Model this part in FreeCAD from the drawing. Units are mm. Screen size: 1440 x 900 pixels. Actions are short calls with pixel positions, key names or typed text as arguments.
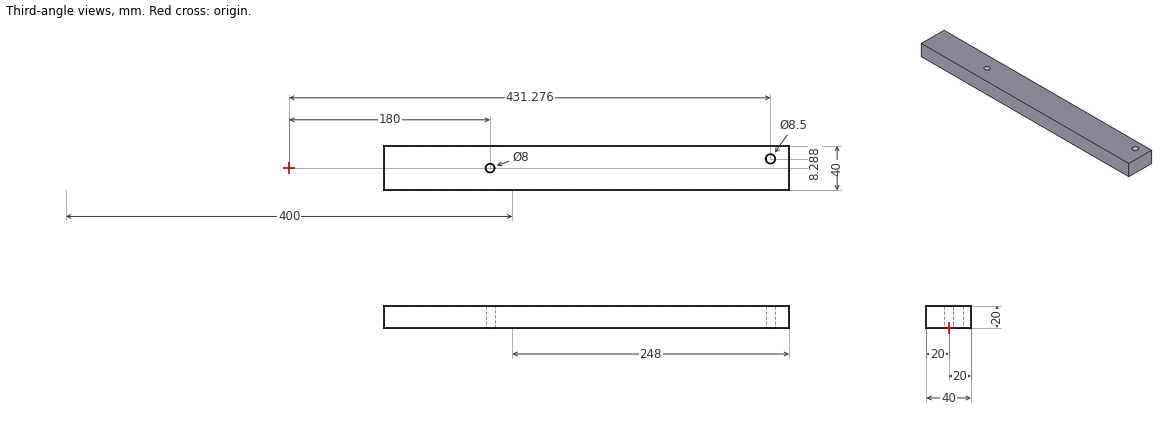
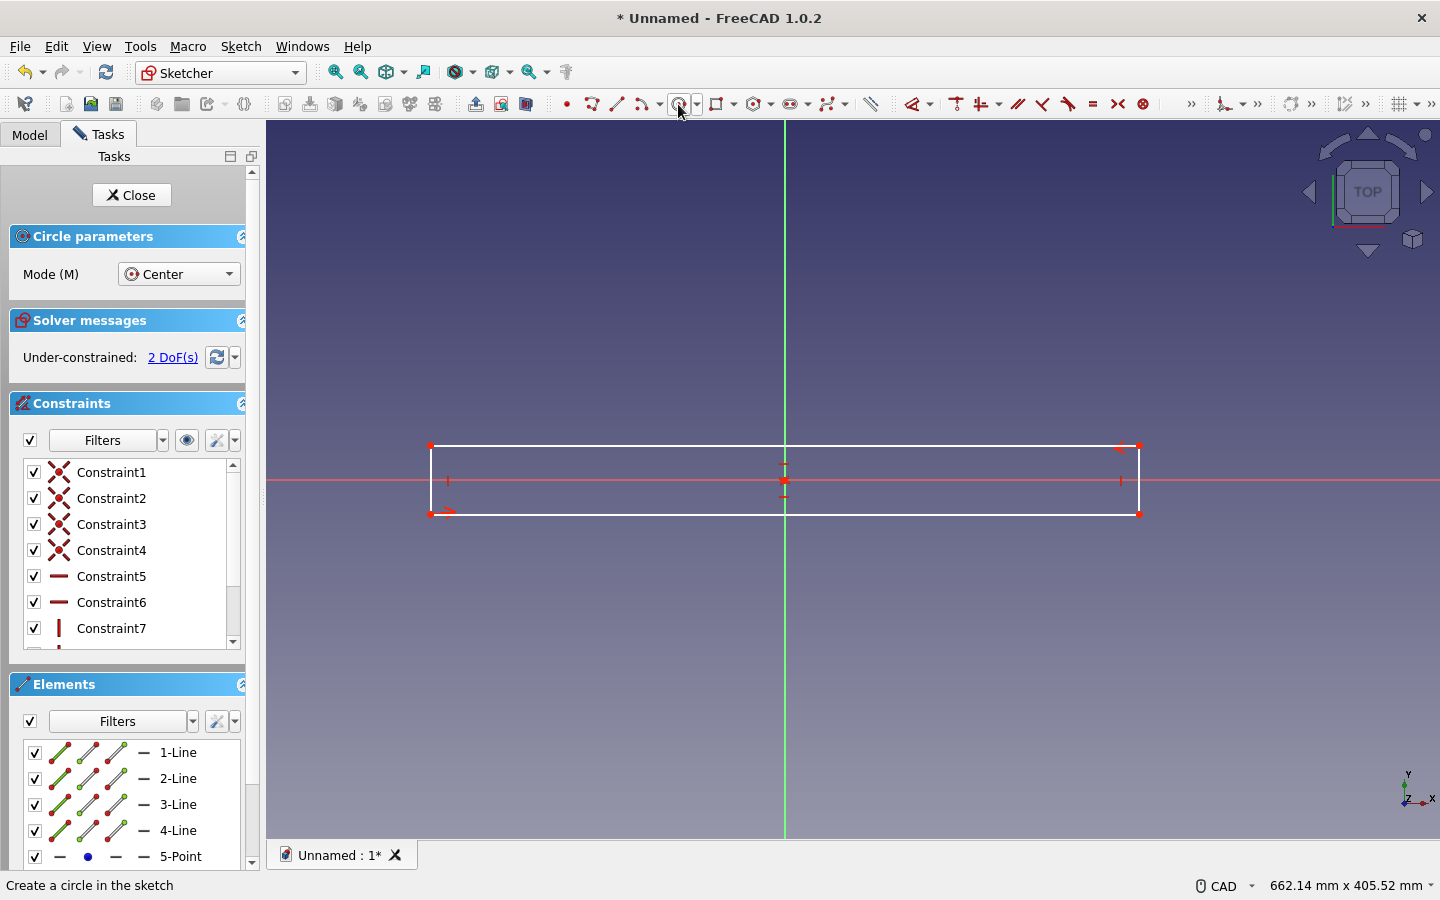
scroll(1104, 480, up, 6)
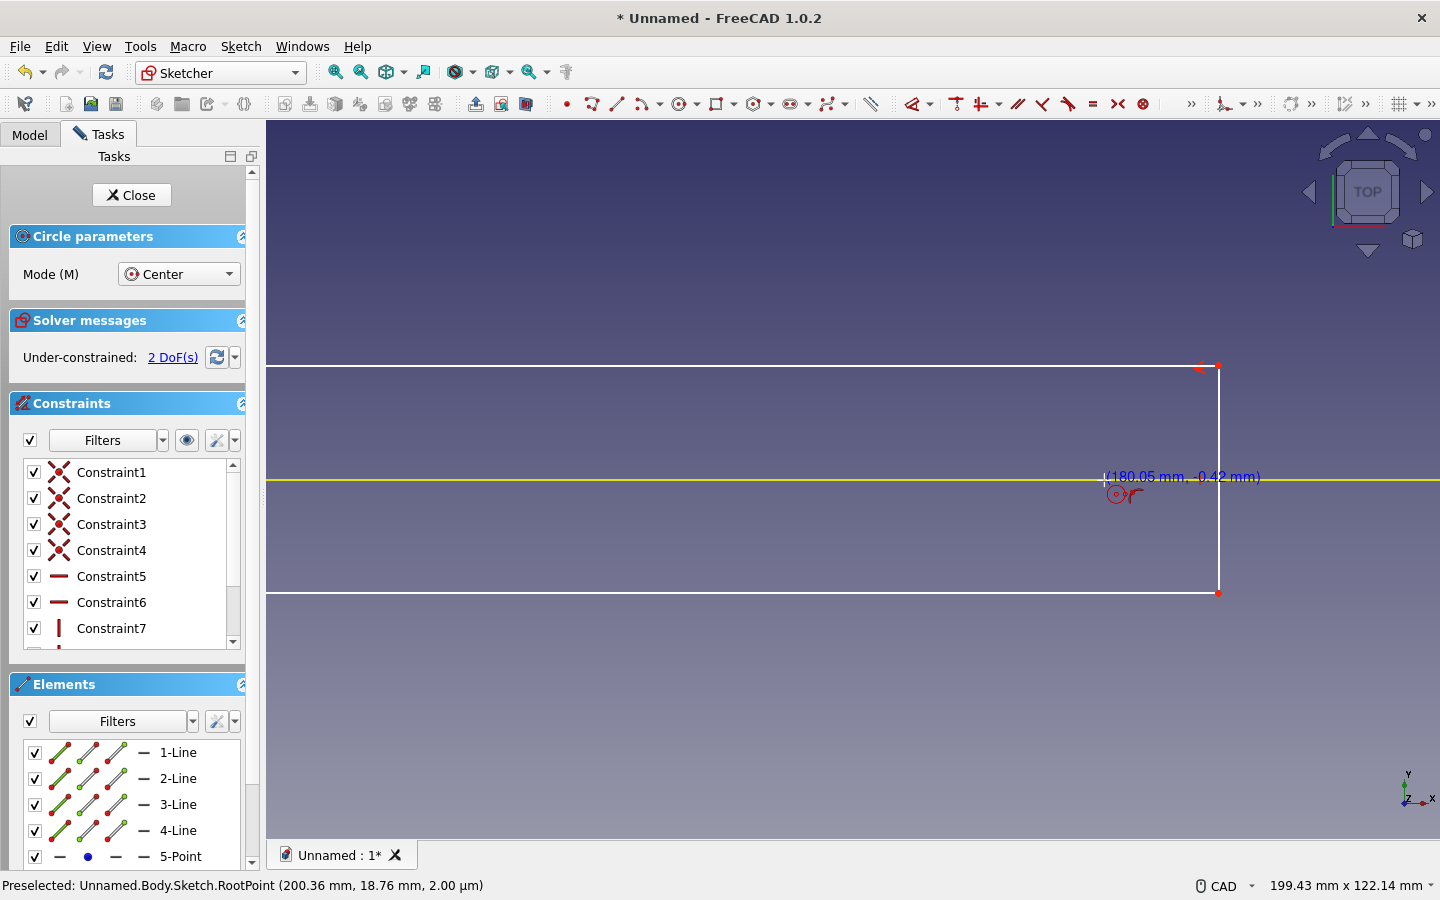
click(1102, 480)
click(1119, 463)
key(Escape)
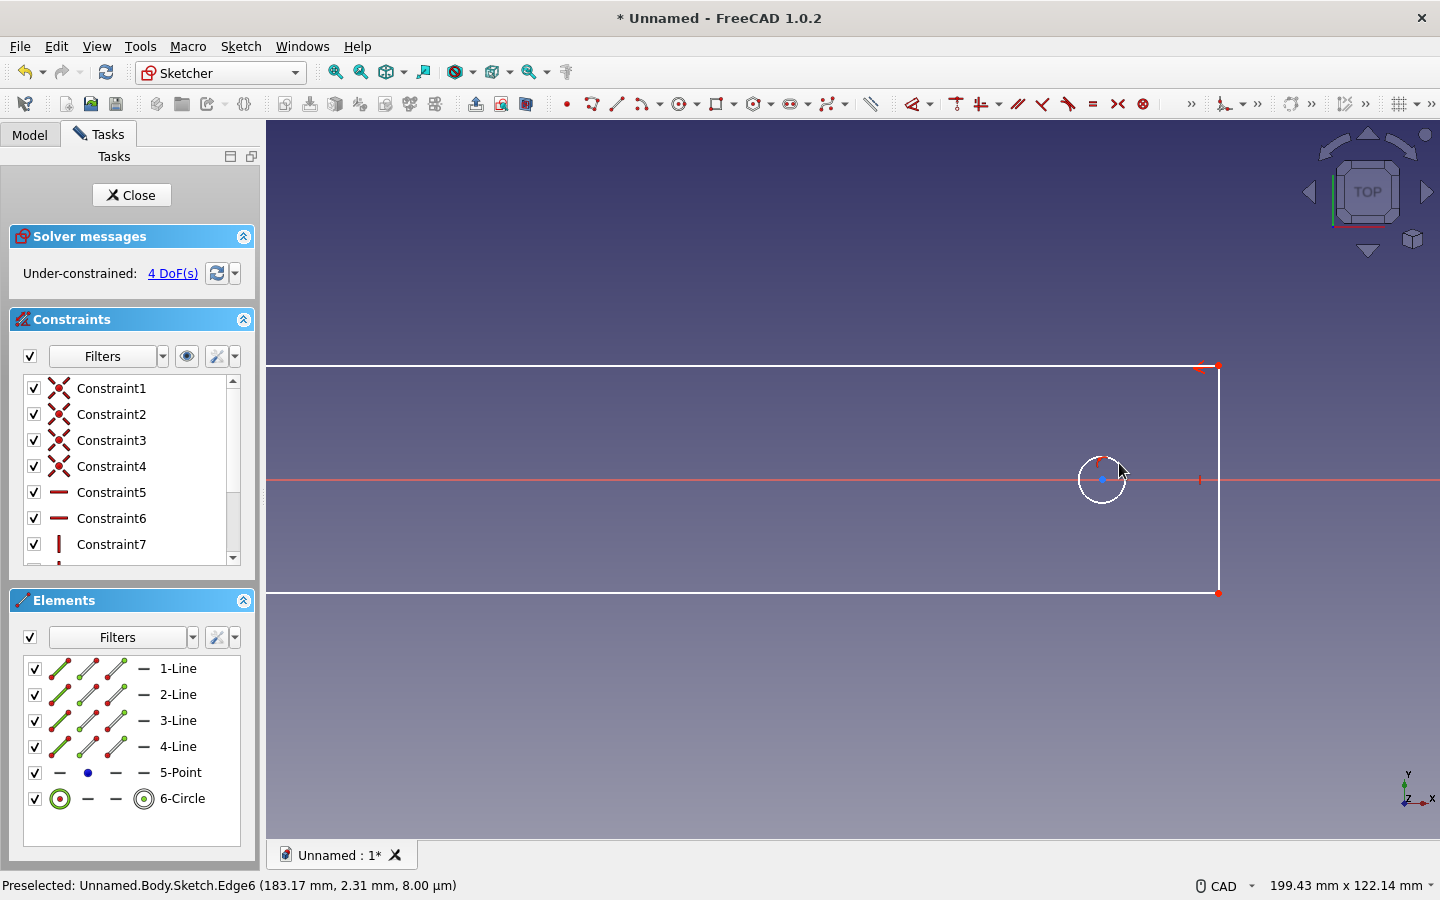
click(1118, 463)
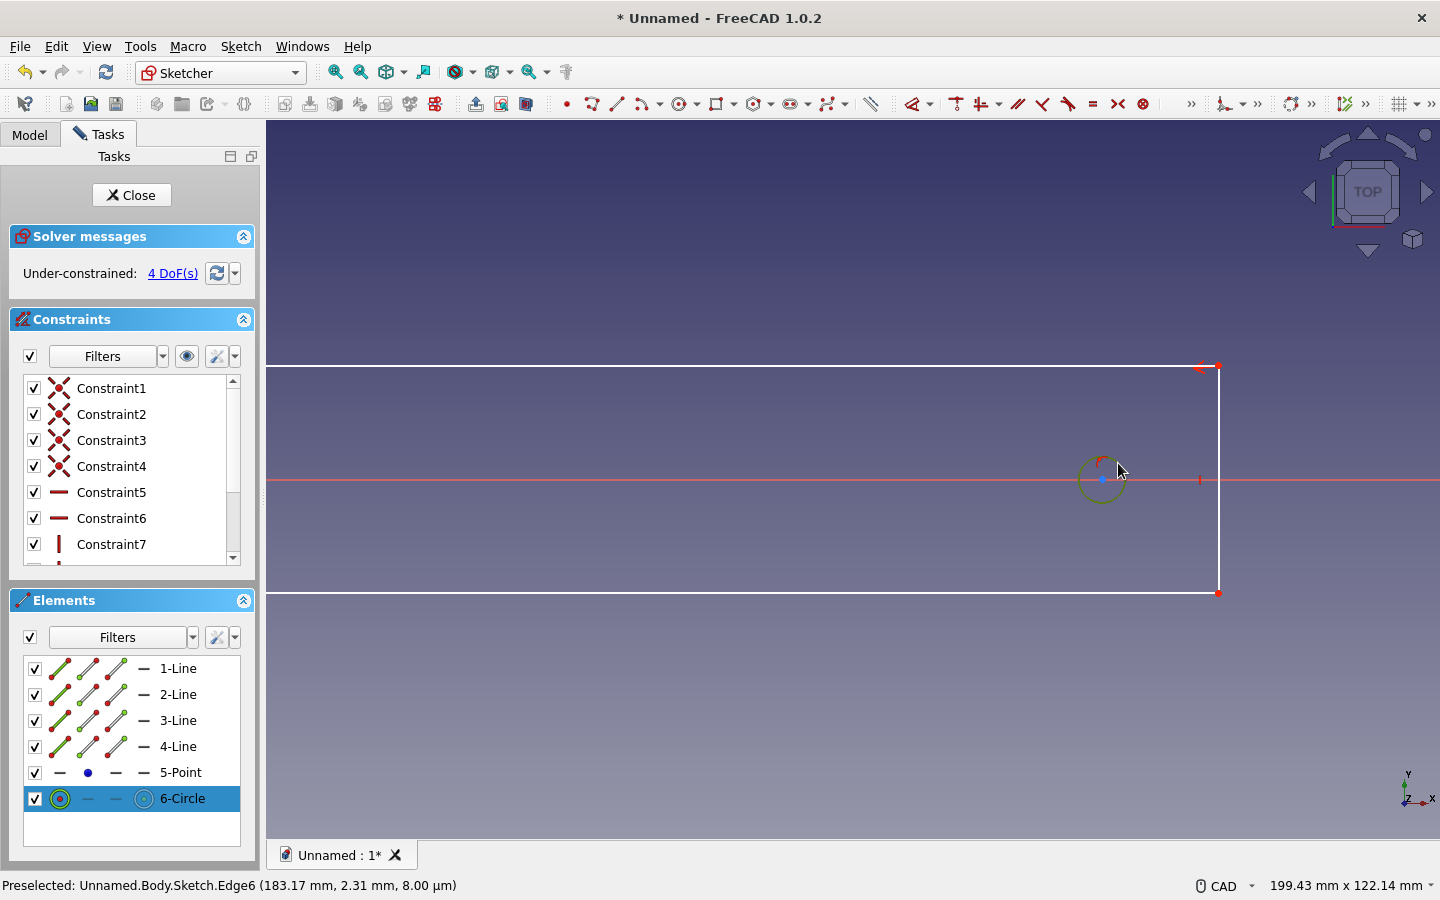
key(k)
key(o)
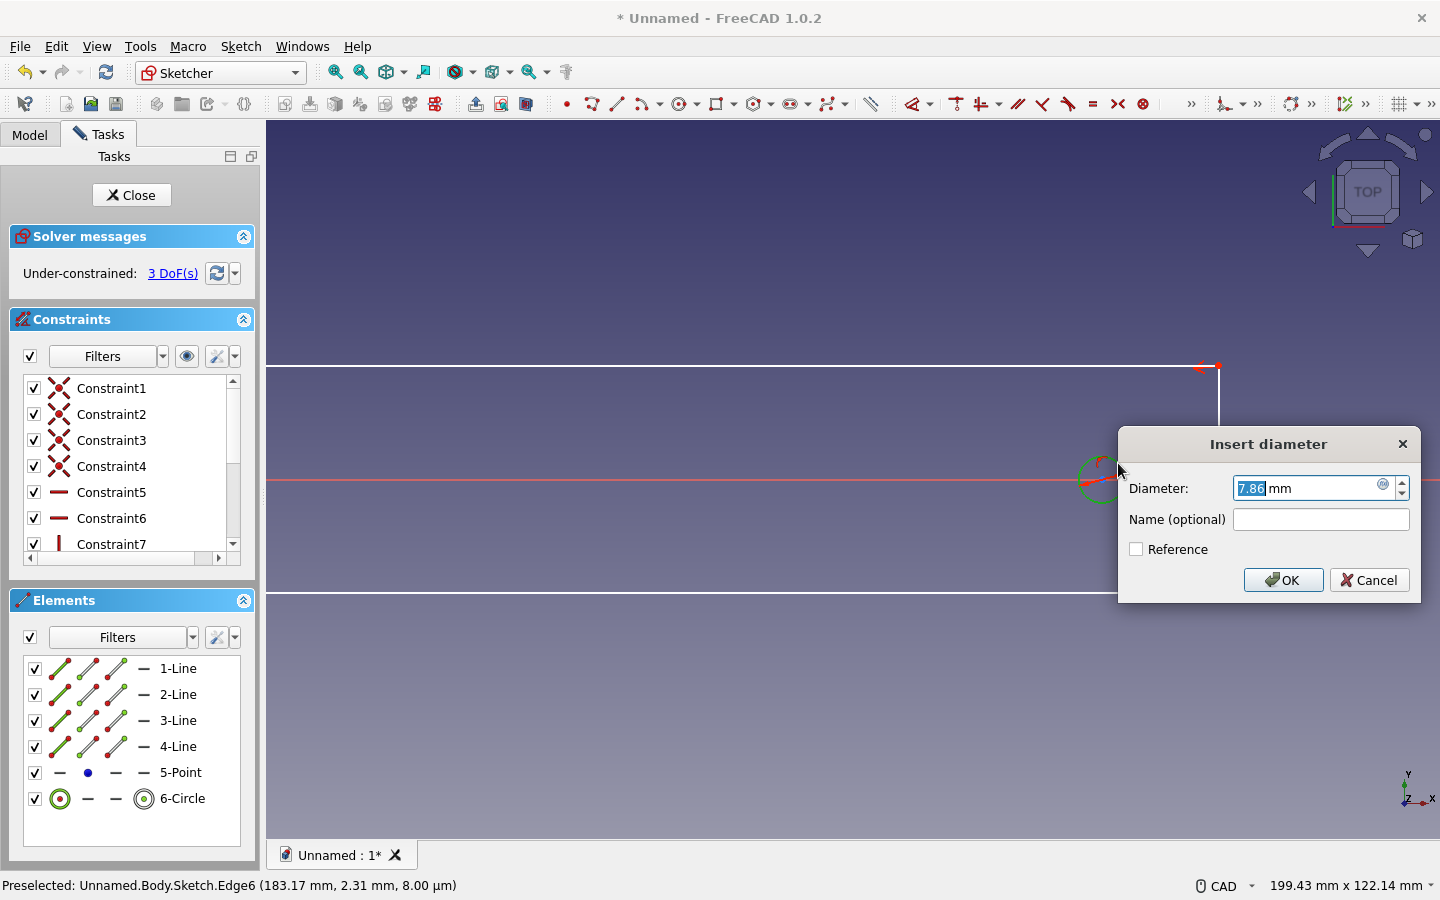
text(8)
key(Return)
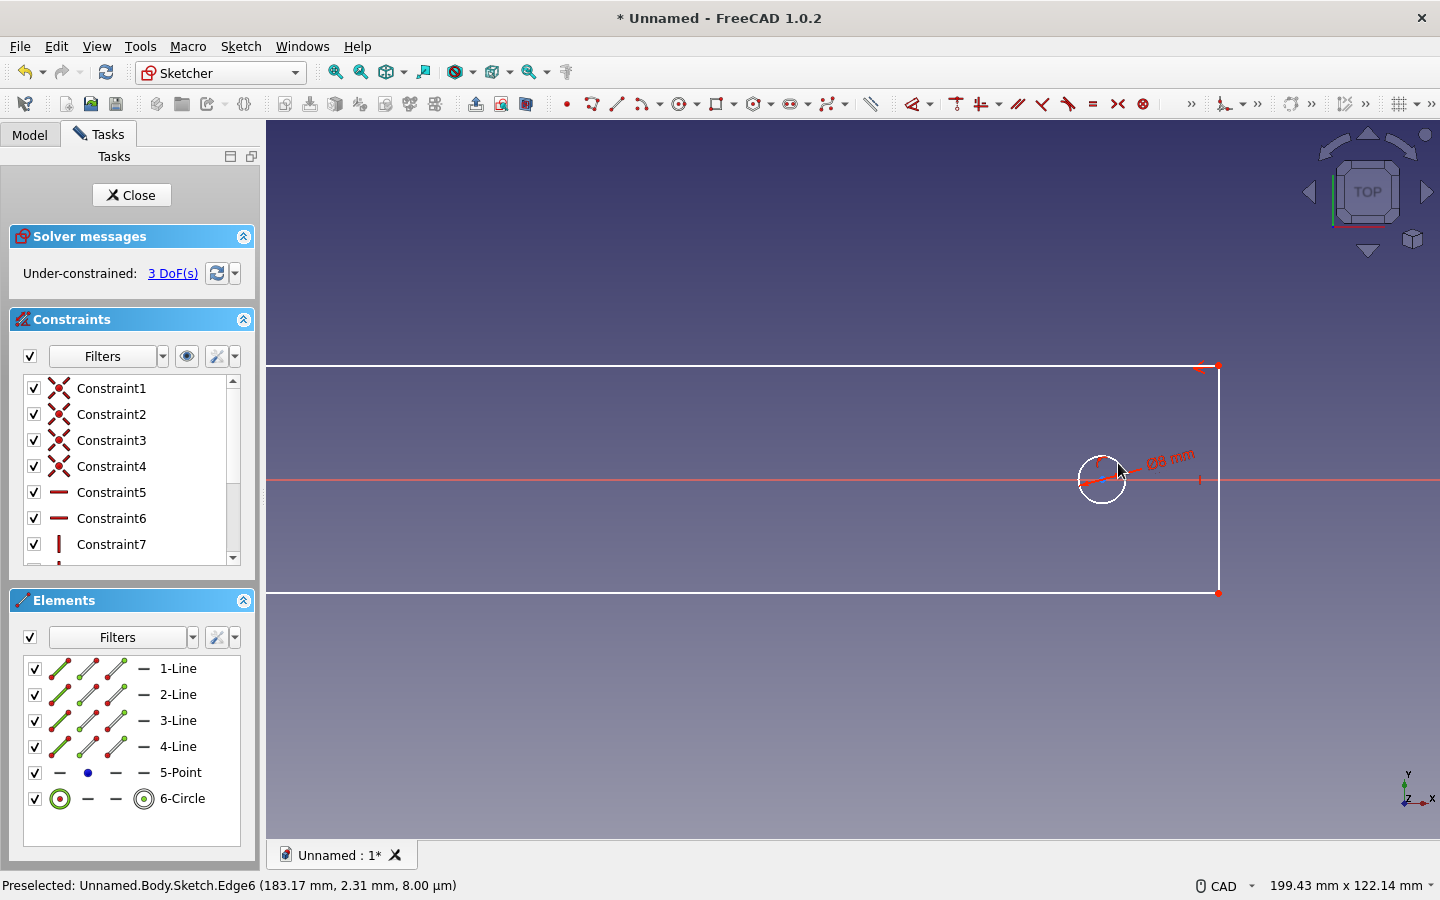
click(1219, 525)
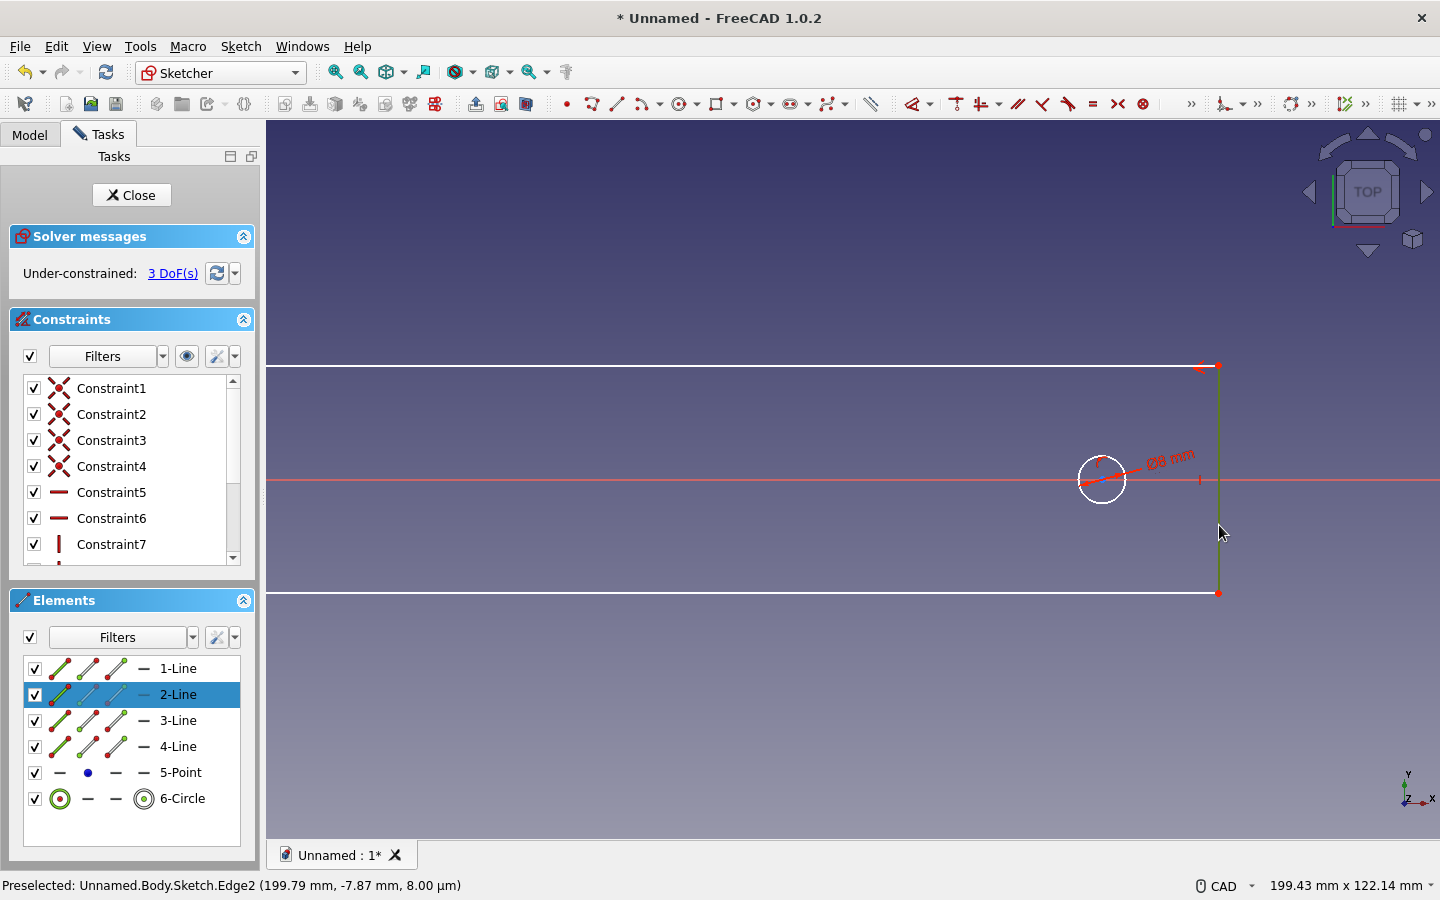
key(i)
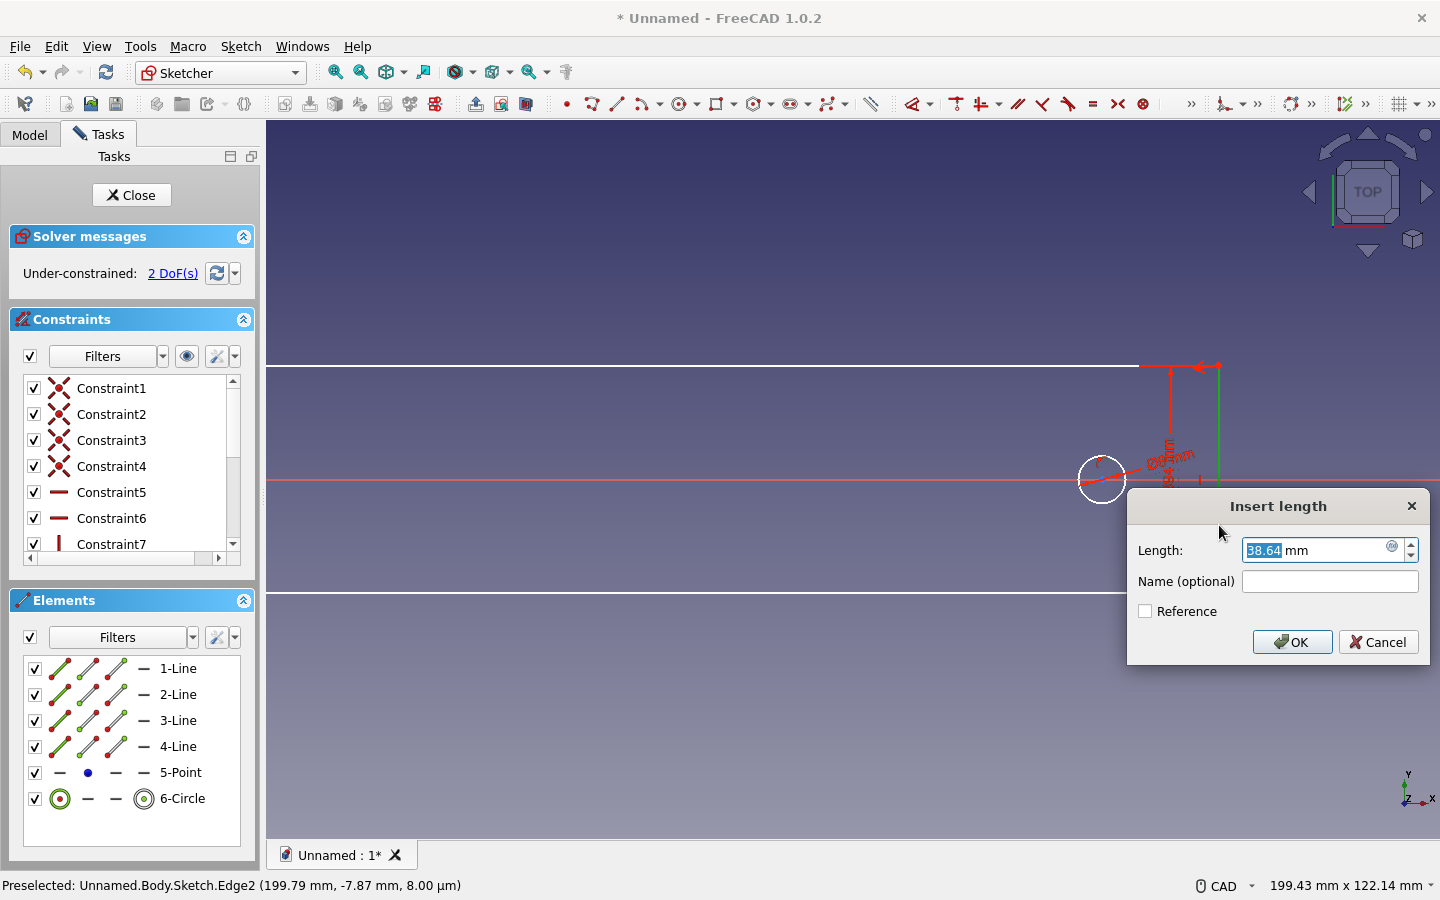
text(40)
key(Return)